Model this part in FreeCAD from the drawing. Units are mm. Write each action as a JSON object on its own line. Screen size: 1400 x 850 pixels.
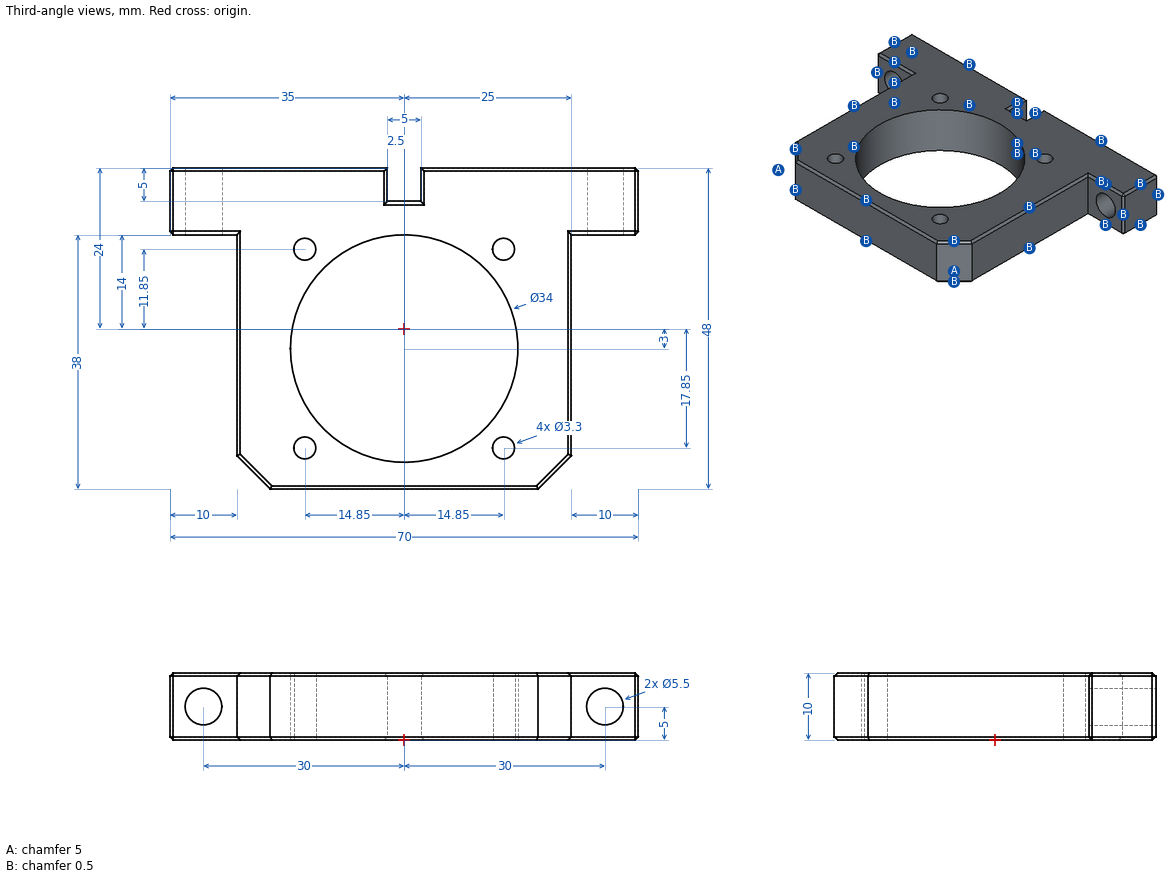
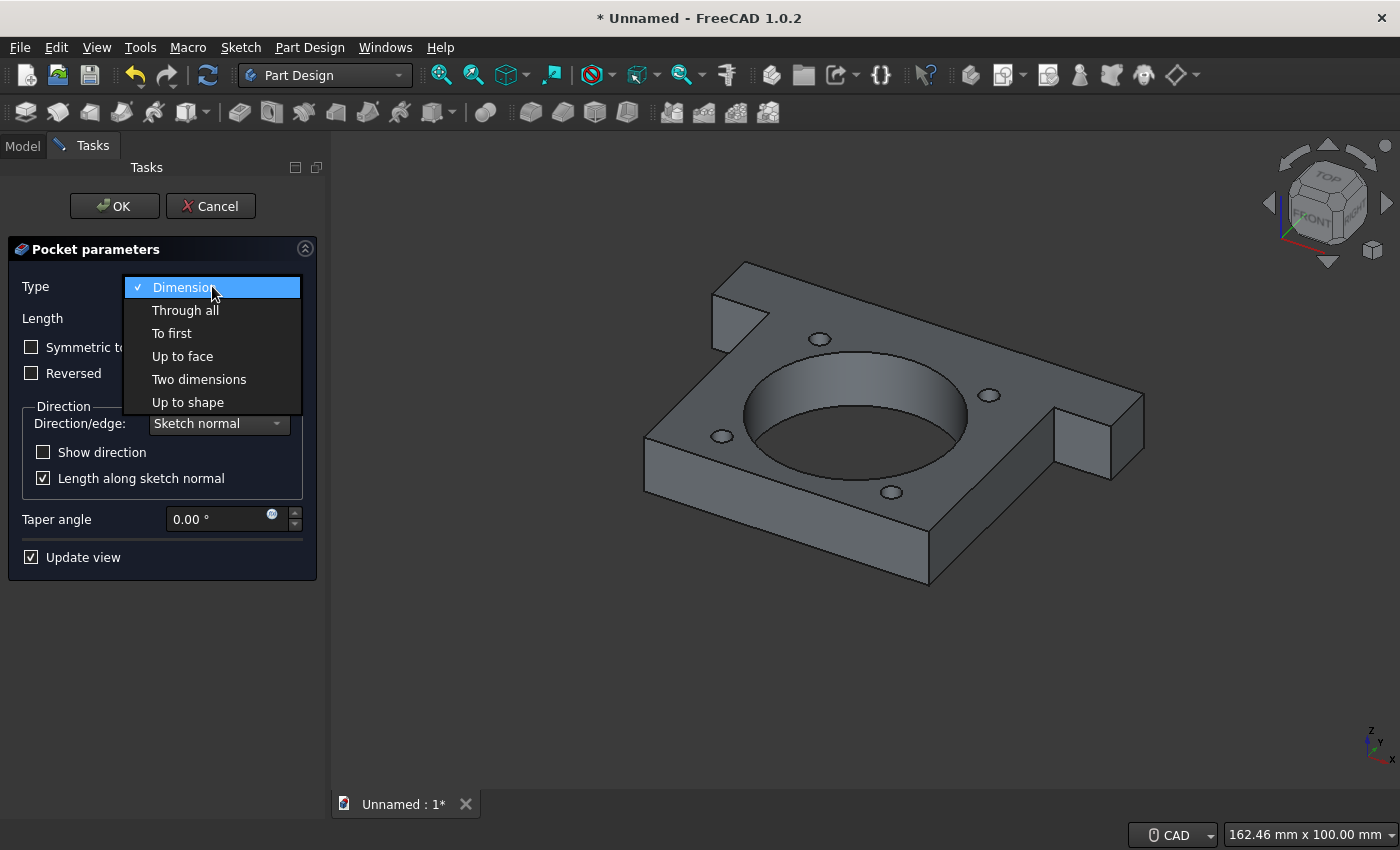
{"action": "left_click", "coordinate": [212, 310]}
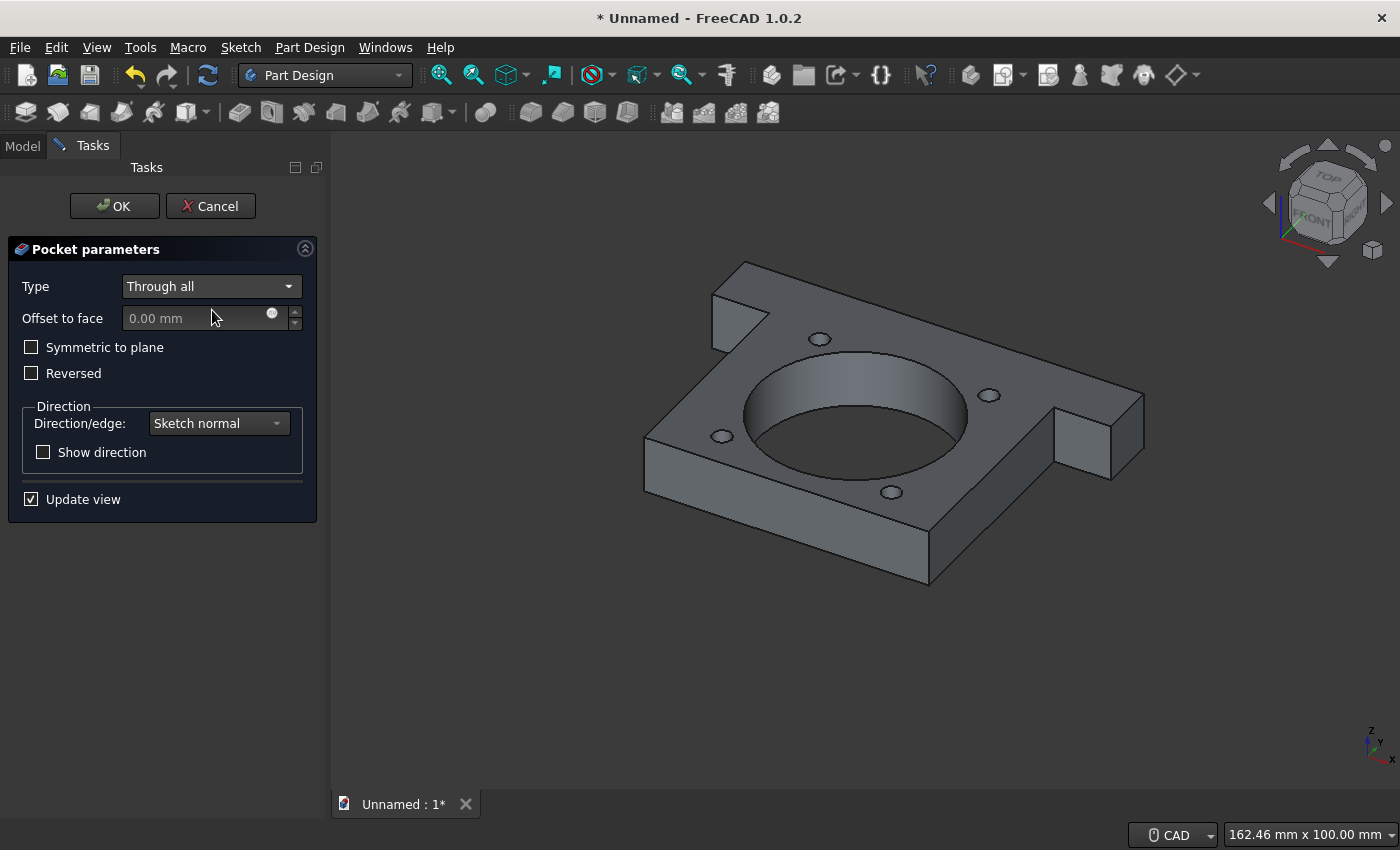
{"action": "left_click", "coordinate": [115, 206]}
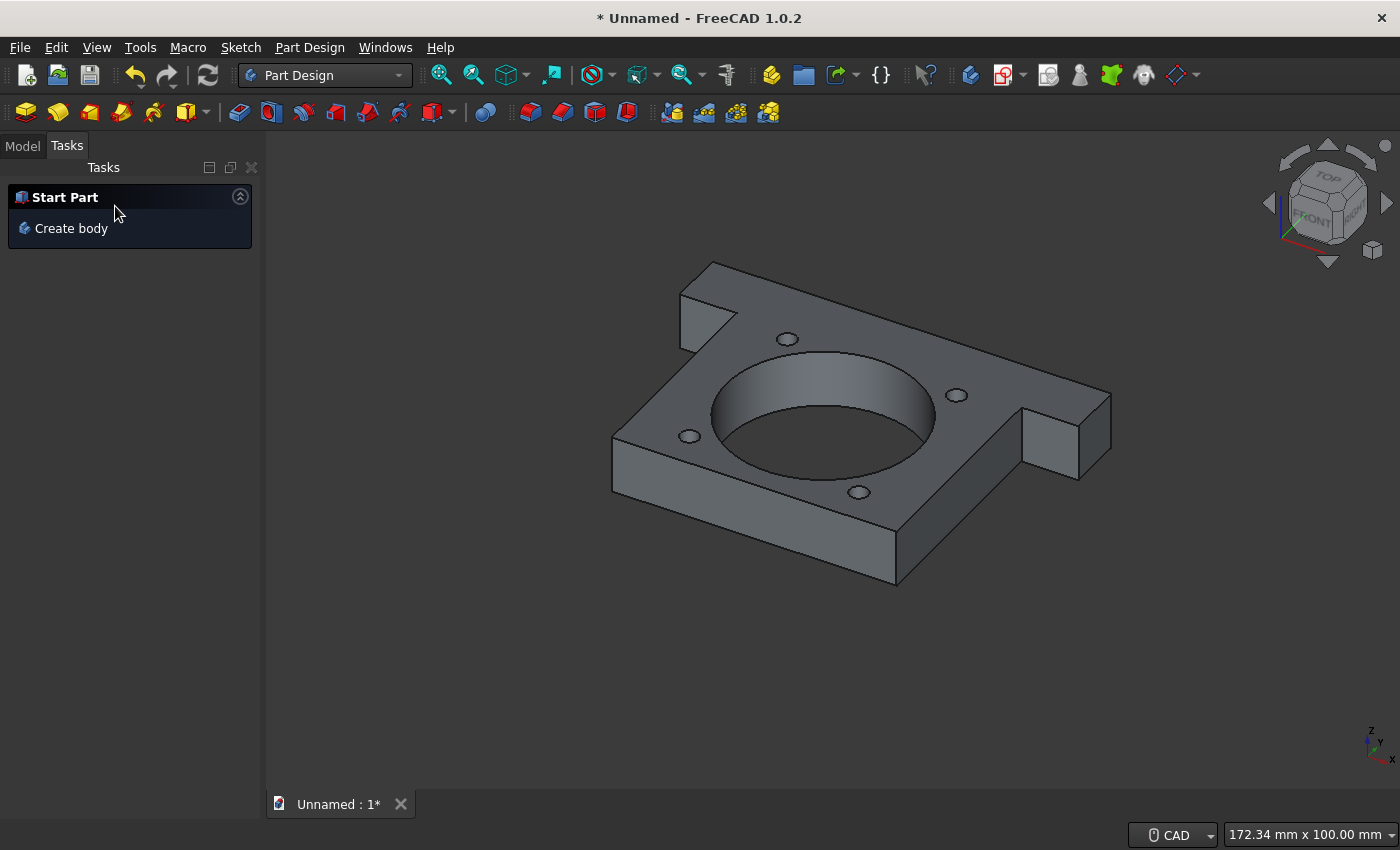
{"action": "left_click", "coordinate": [1050, 443]}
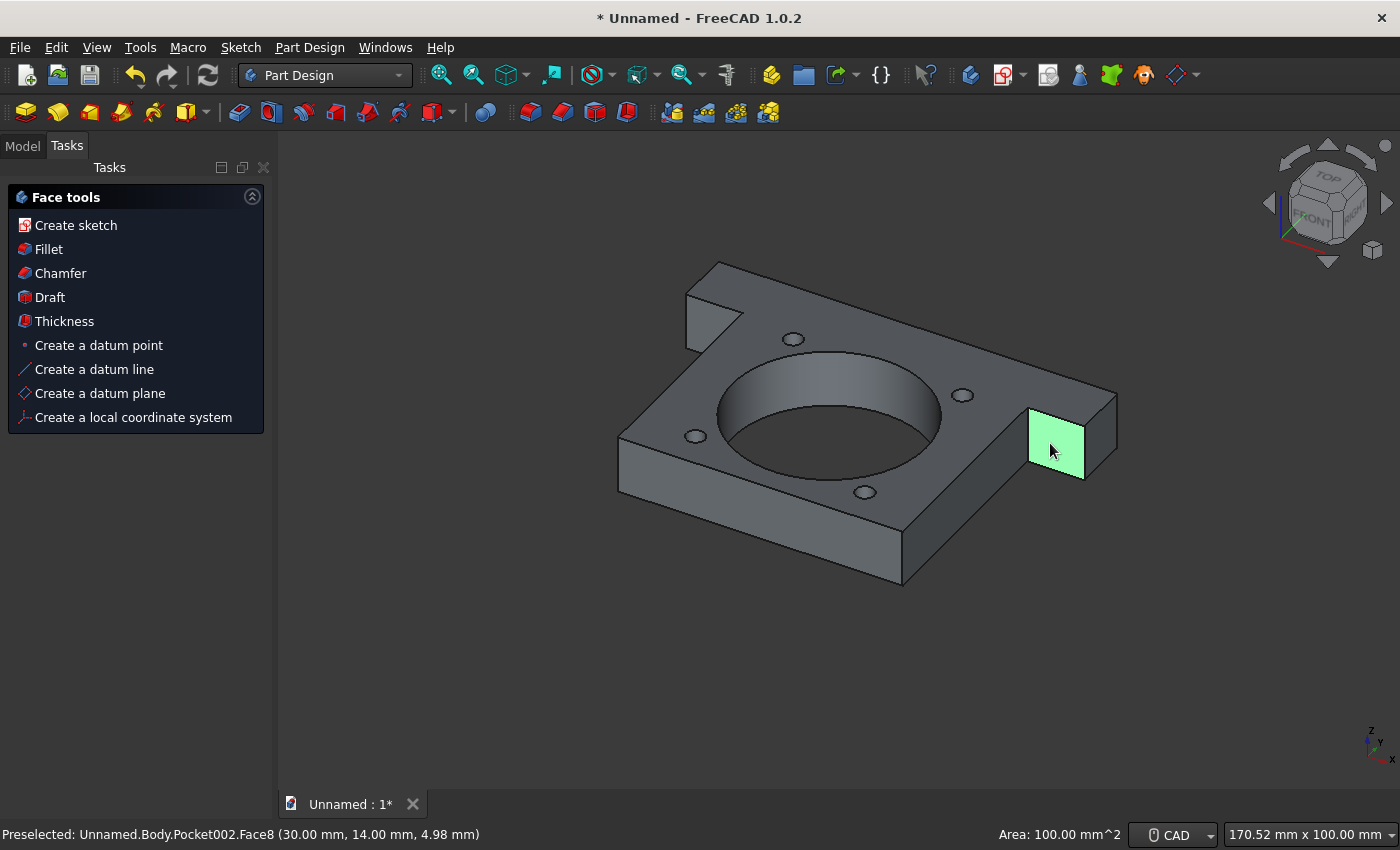
{"action": "left_click", "coordinate": [1004, 76]}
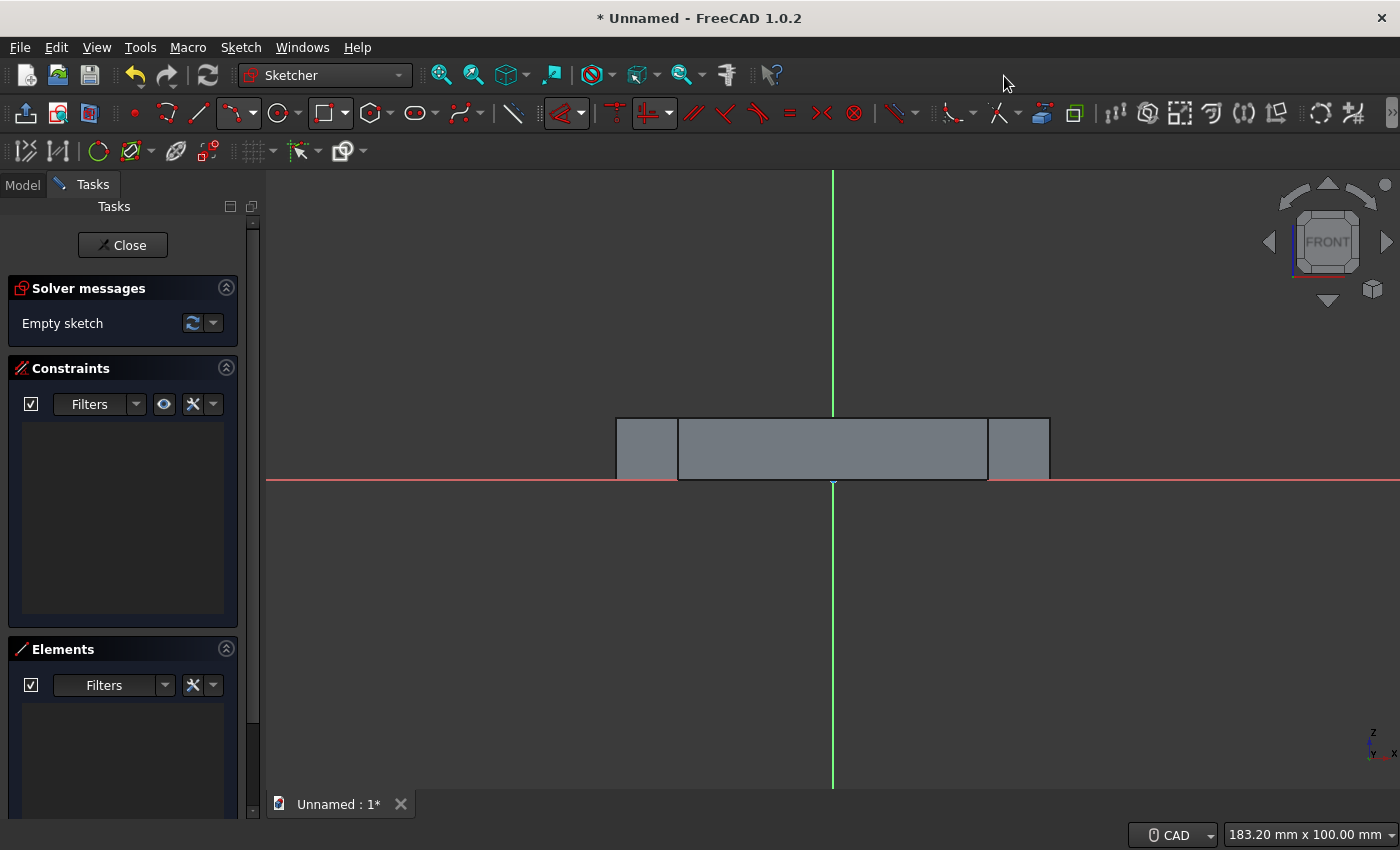
{"action": "scroll", "coordinate": [972, 407], "scroll_direction": "up", "scroll_amount": 2}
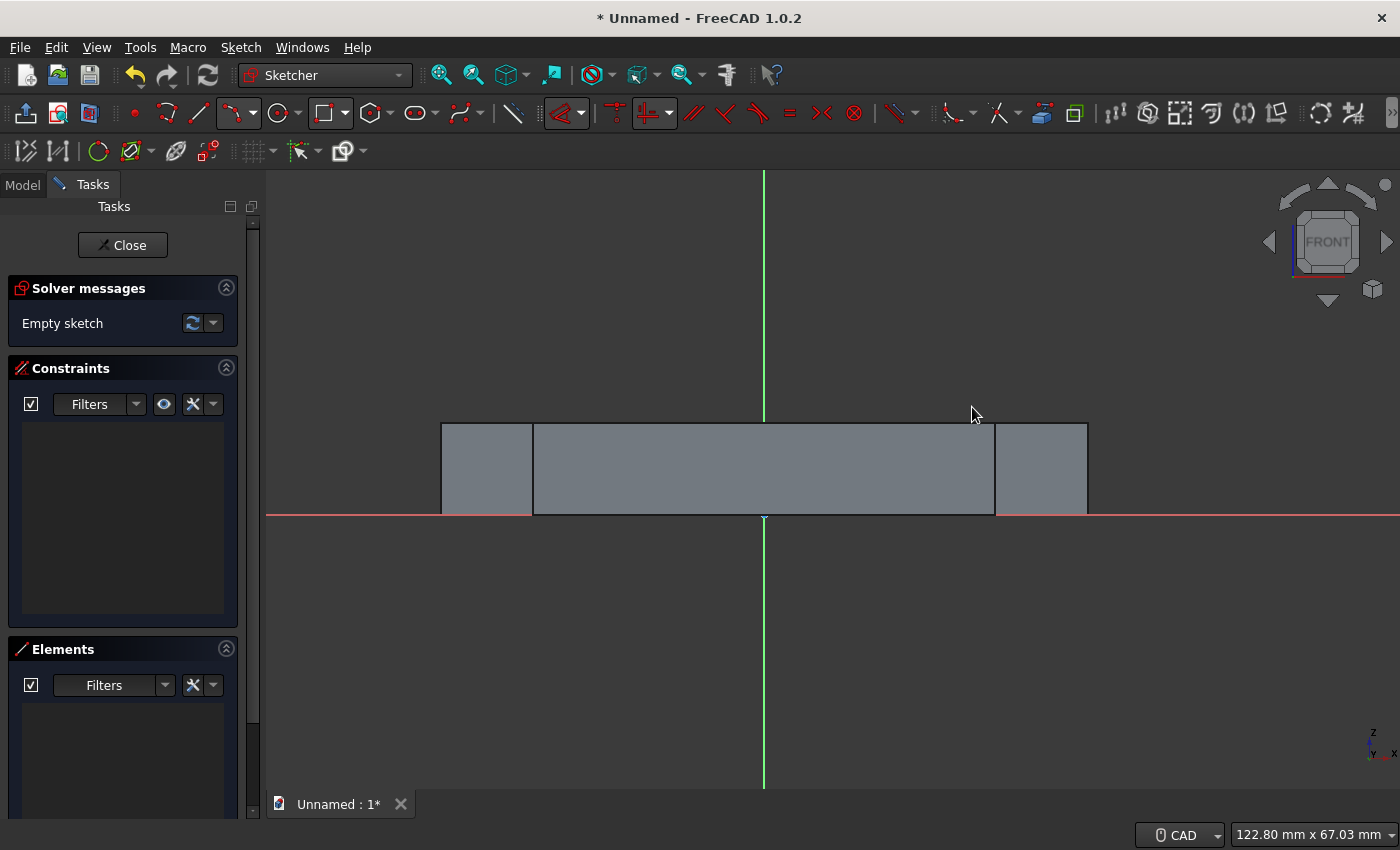
{"action": "left_click", "coordinate": [278, 114]}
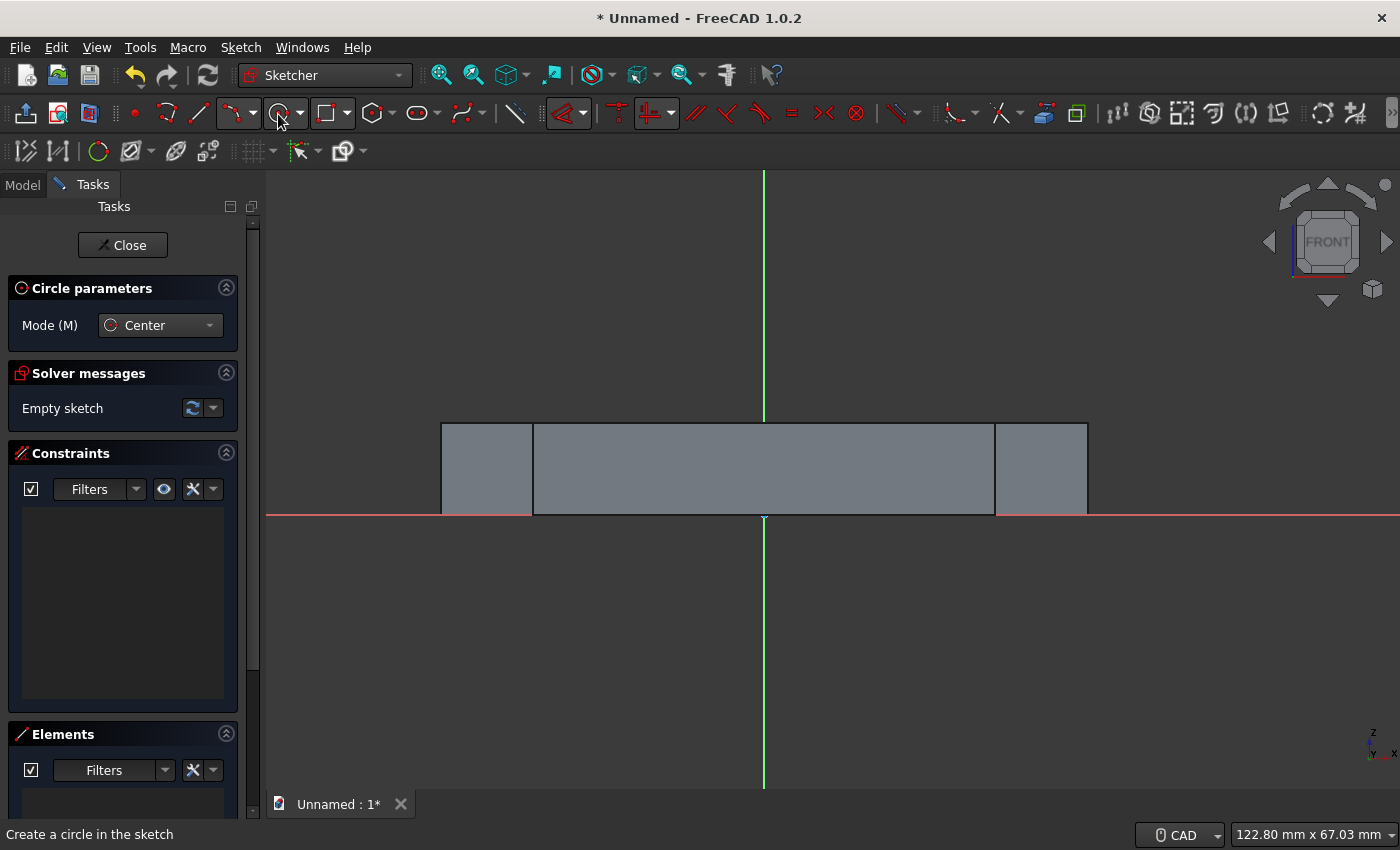
{"action": "left_click", "coordinate": [1041, 469]}
{"action": "left_click", "coordinate": [1059, 451]}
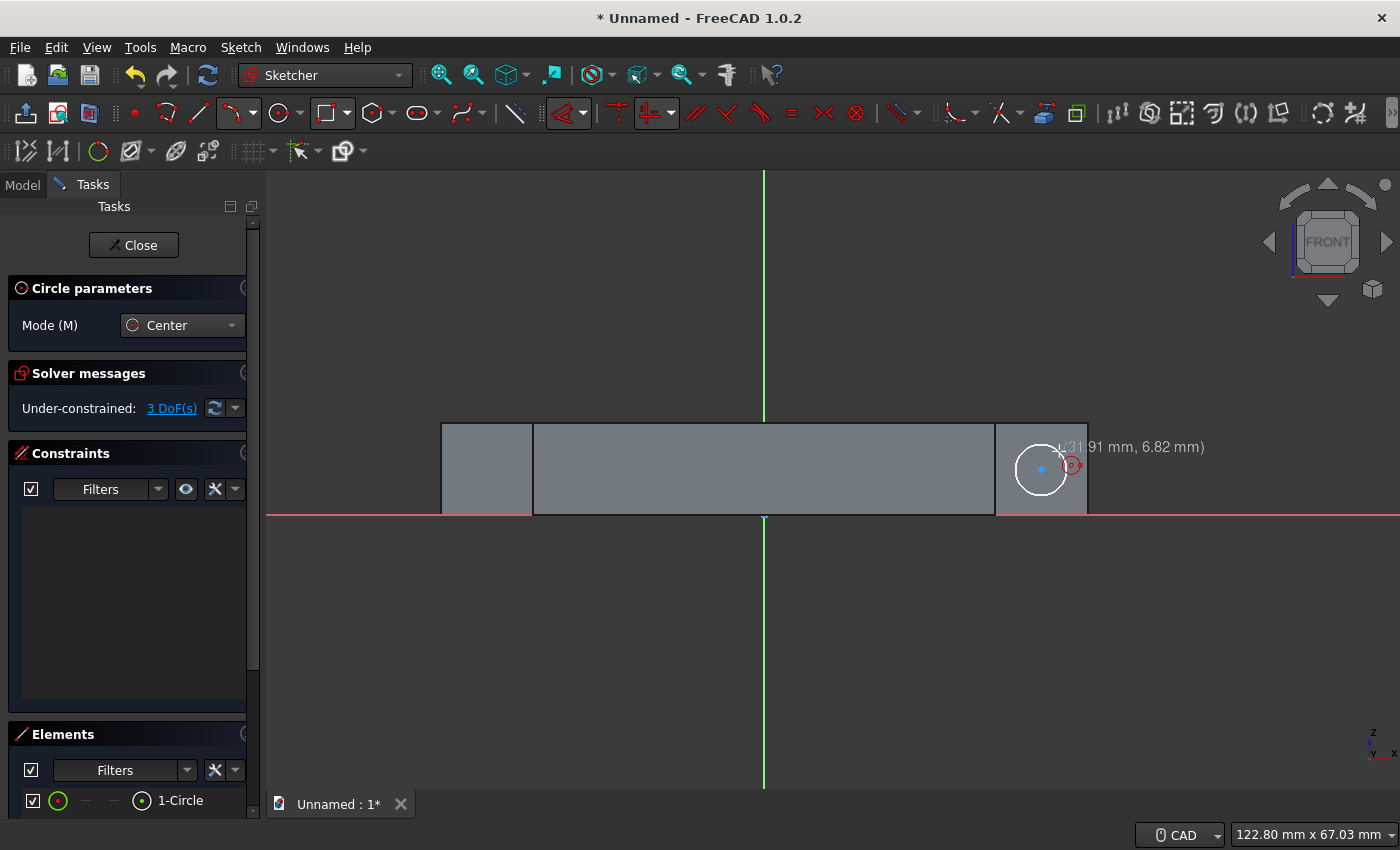
{"action": "left_click", "coordinate": [487, 469]}
{"action": "left_click", "coordinate": [505, 451]}
{"action": "key", "text": "Escape"}